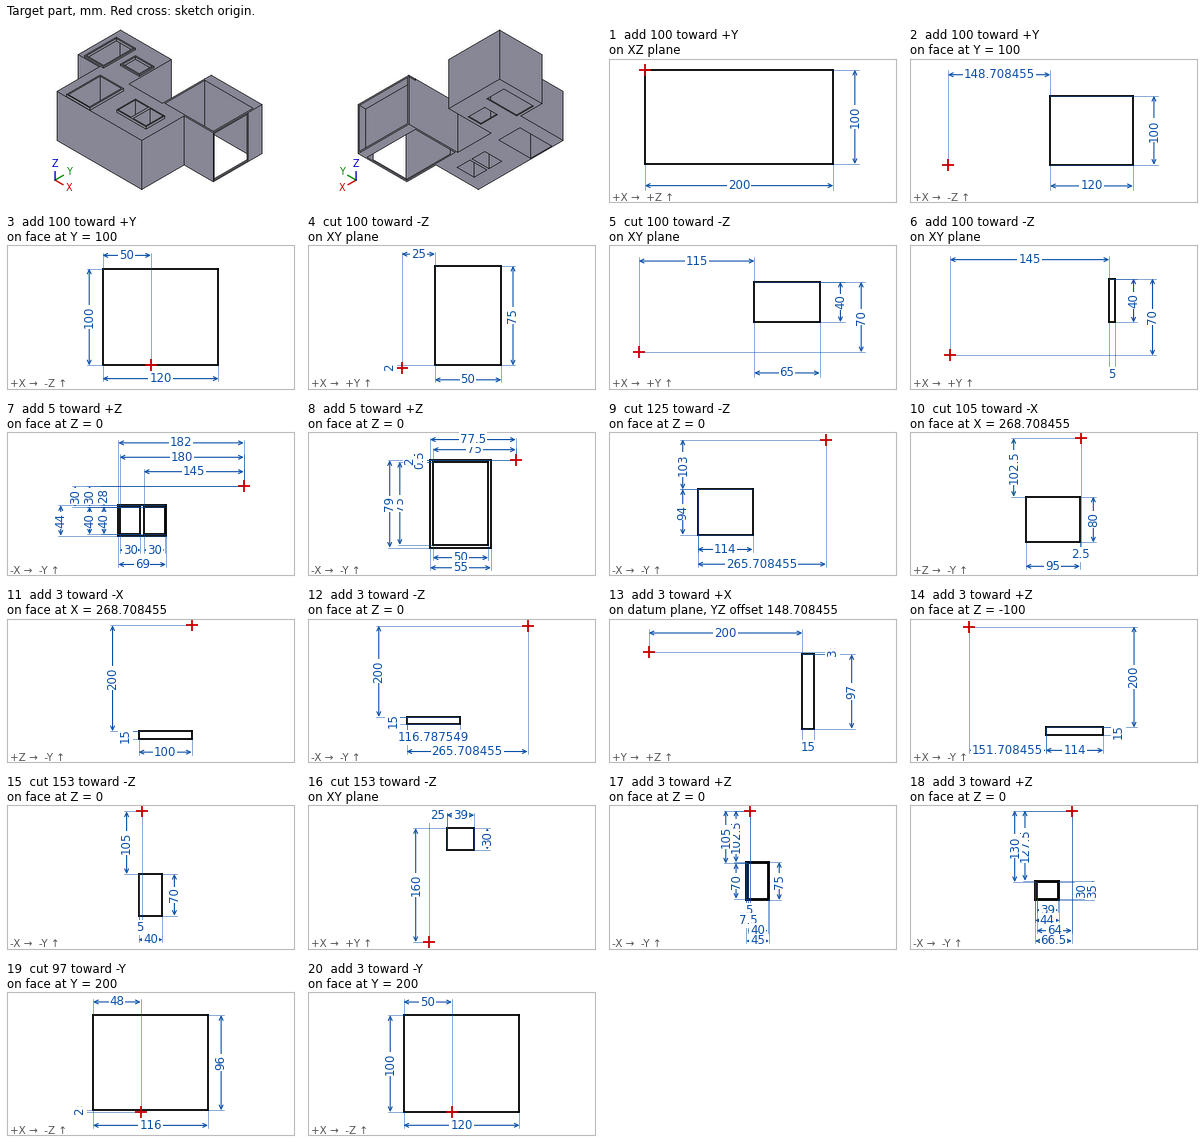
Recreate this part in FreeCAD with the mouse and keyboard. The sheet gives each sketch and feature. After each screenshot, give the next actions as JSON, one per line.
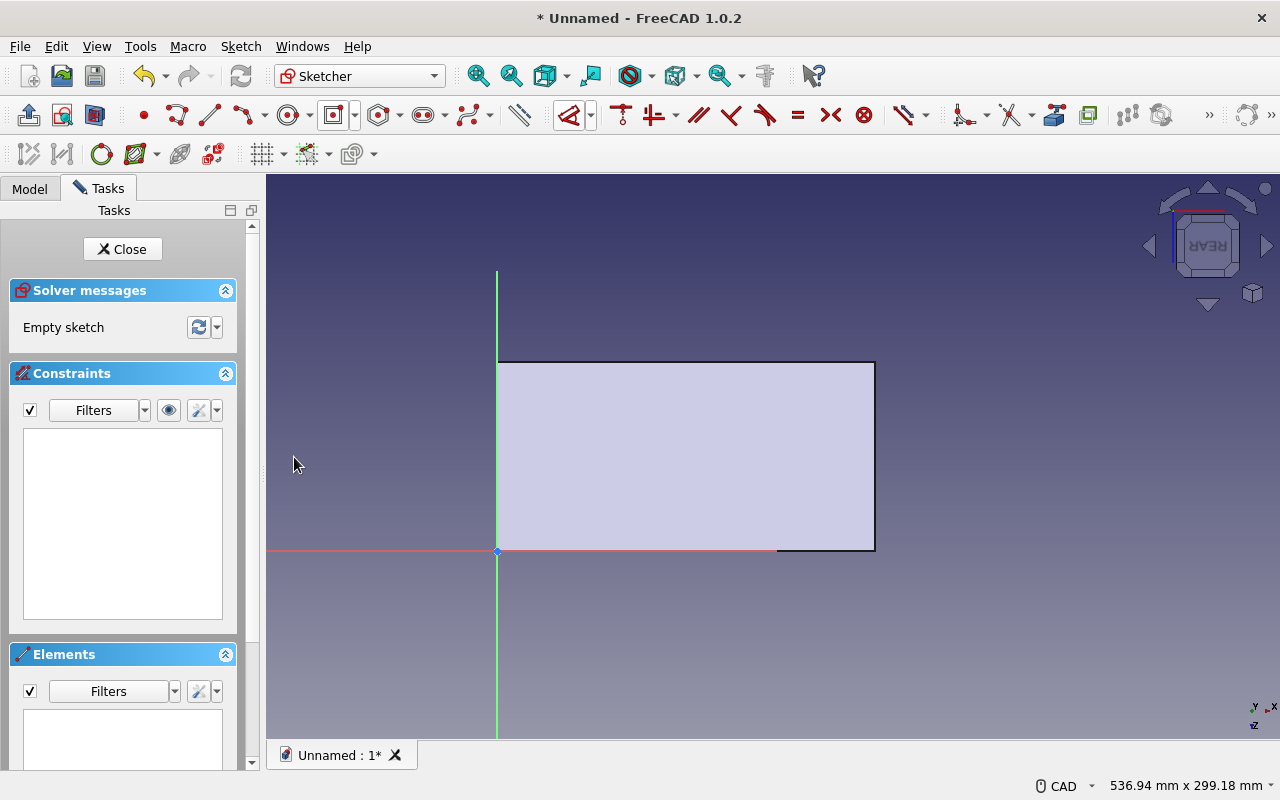
{"action": "key", "text": "g r"}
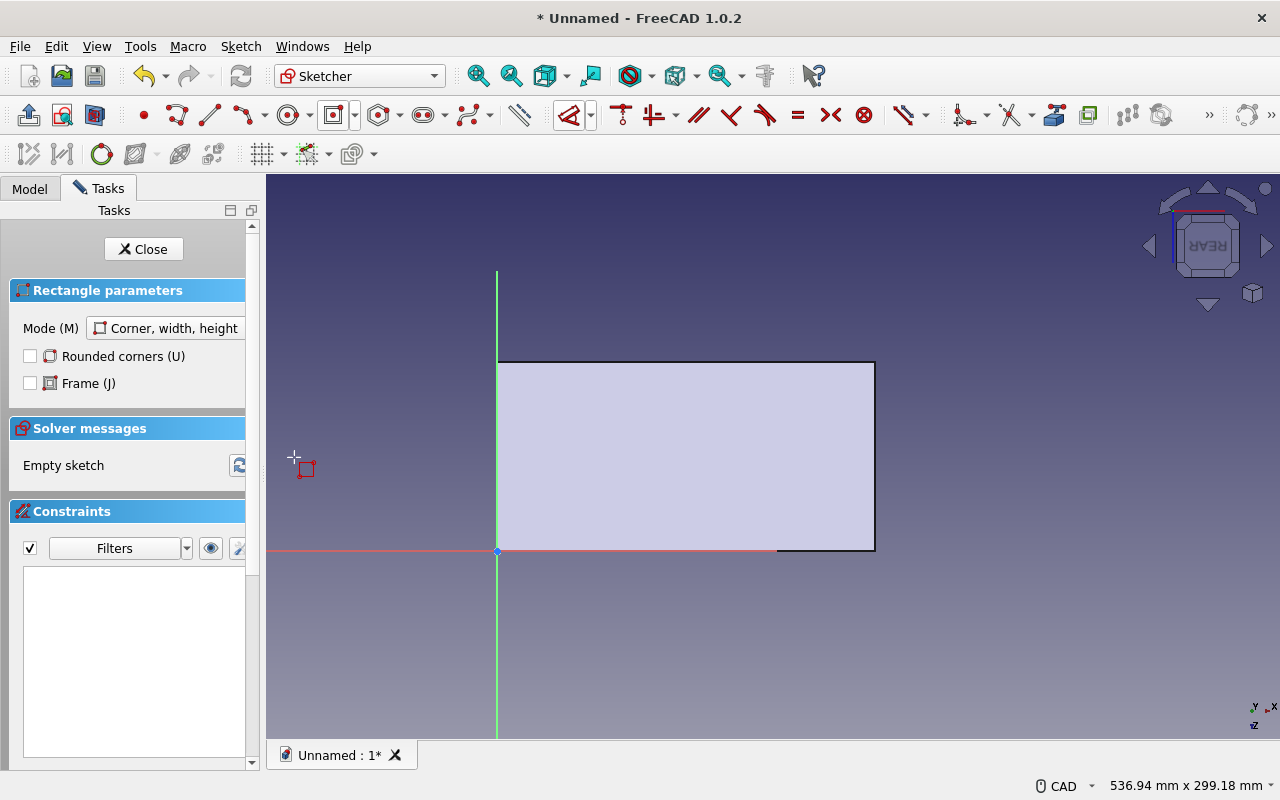
{"action": "left_click", "coordinate": [778, 362]}
{"action": "left_click", "coordinate": [1005, 551]}
{"action": "key", "text": "Escape"}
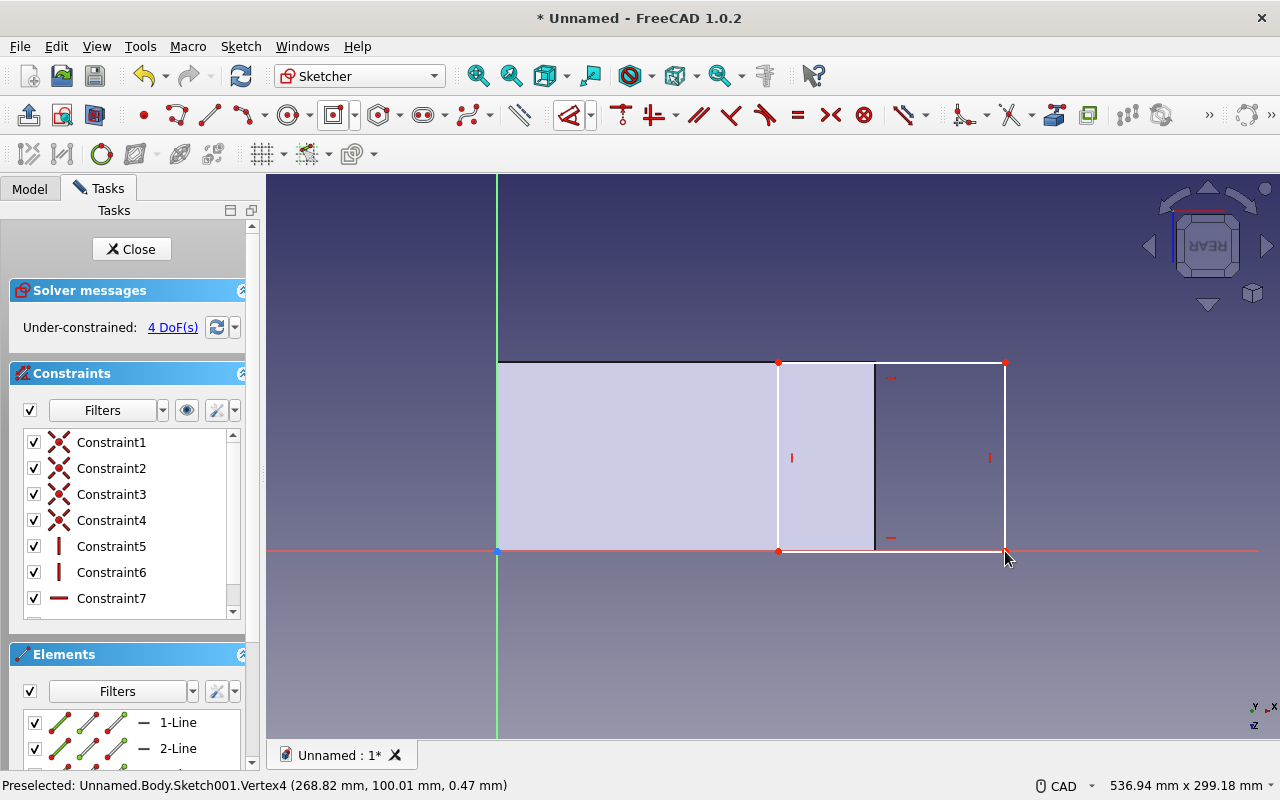
{"action": "left_click", "coordinate": [778, 552]}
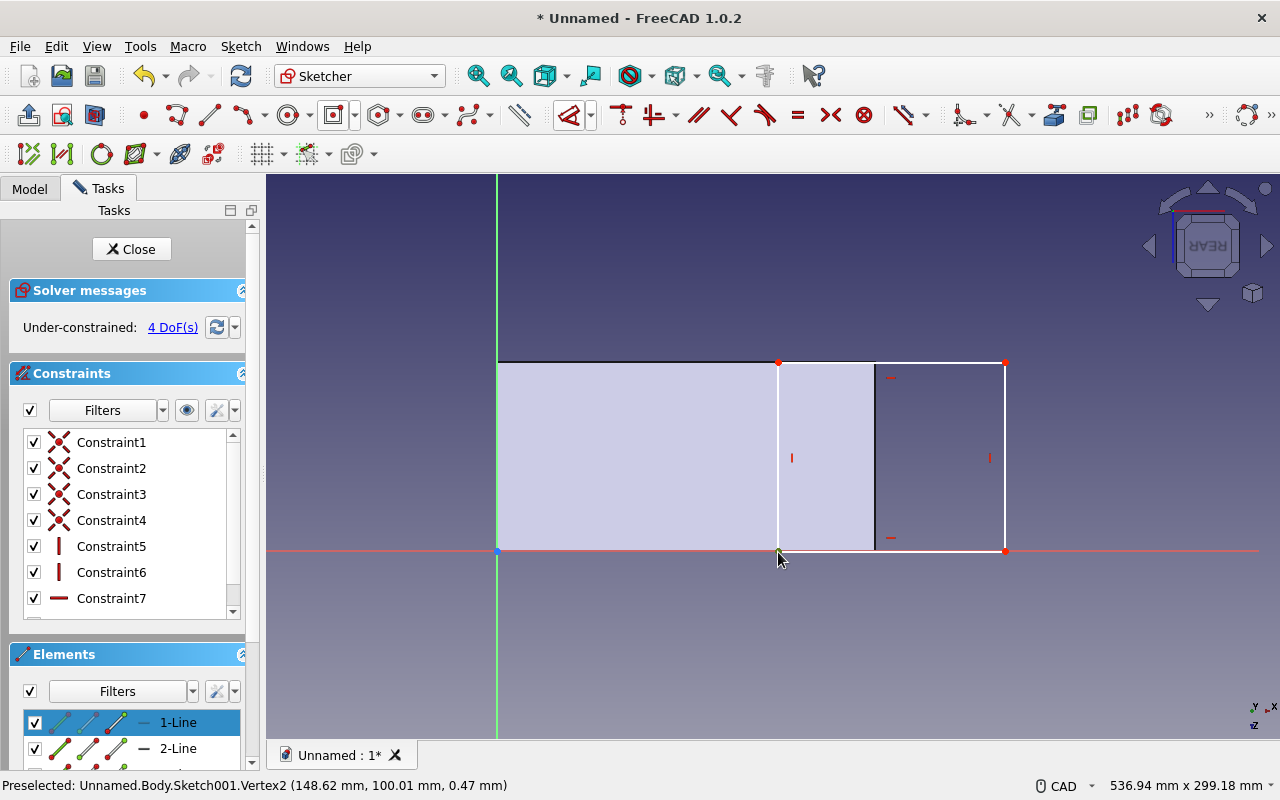
{"action": "left_click", "coordinate": [353, 551]}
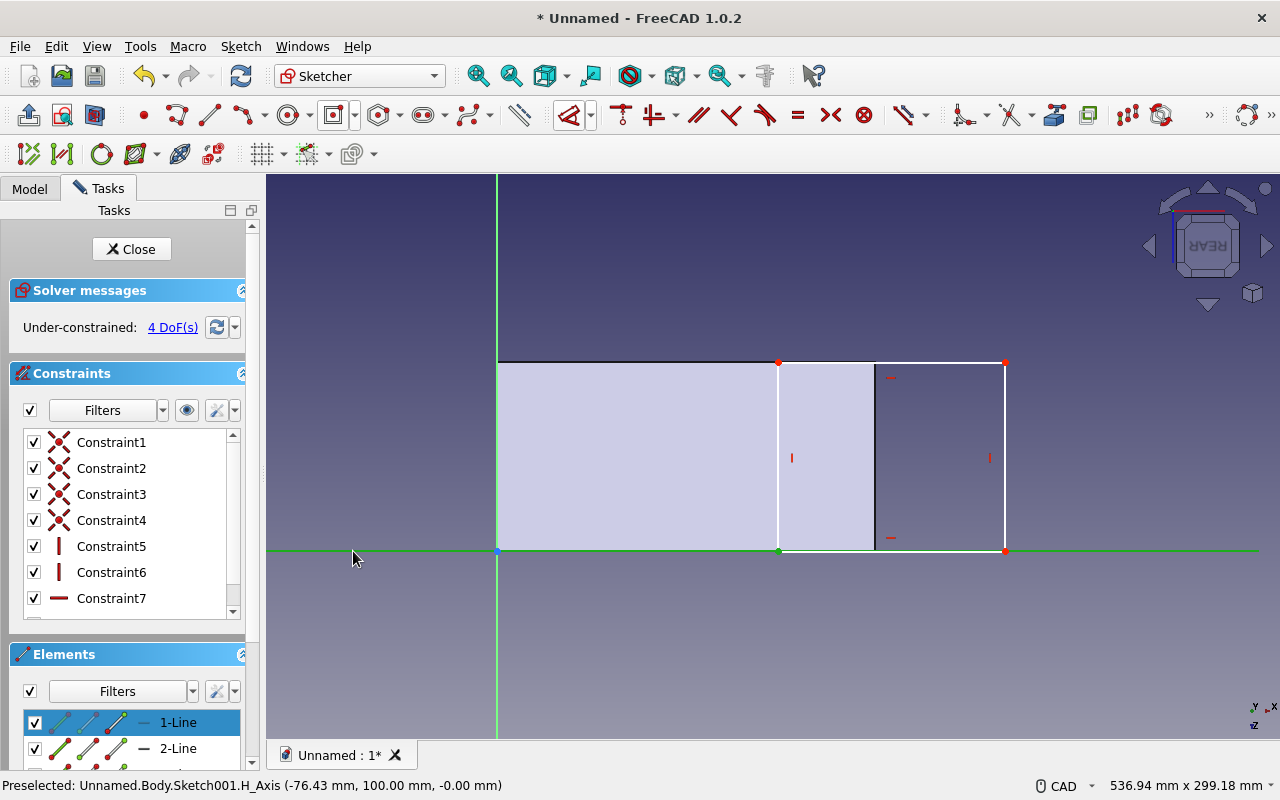
{"action": "left_click", "coordinate": [621, 116]}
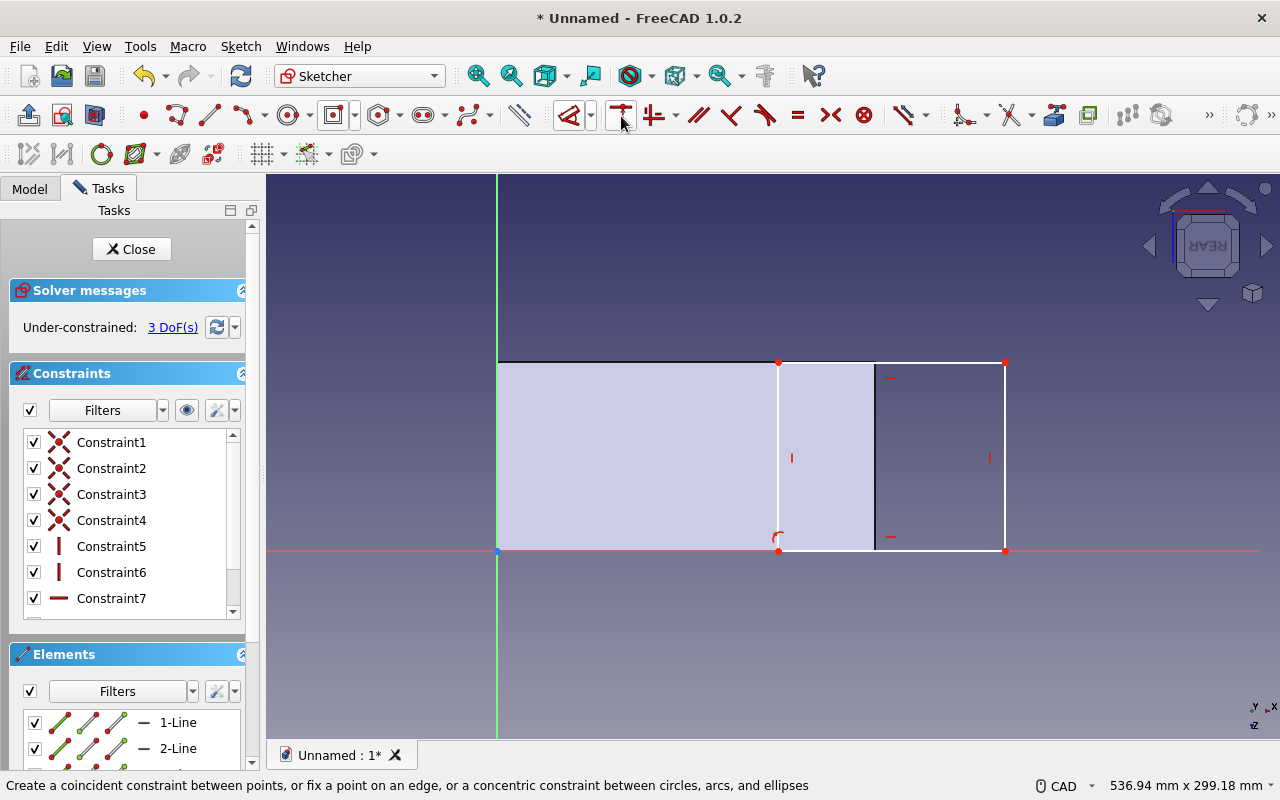
{"action": "left_click", "coordinate": [568, 116]}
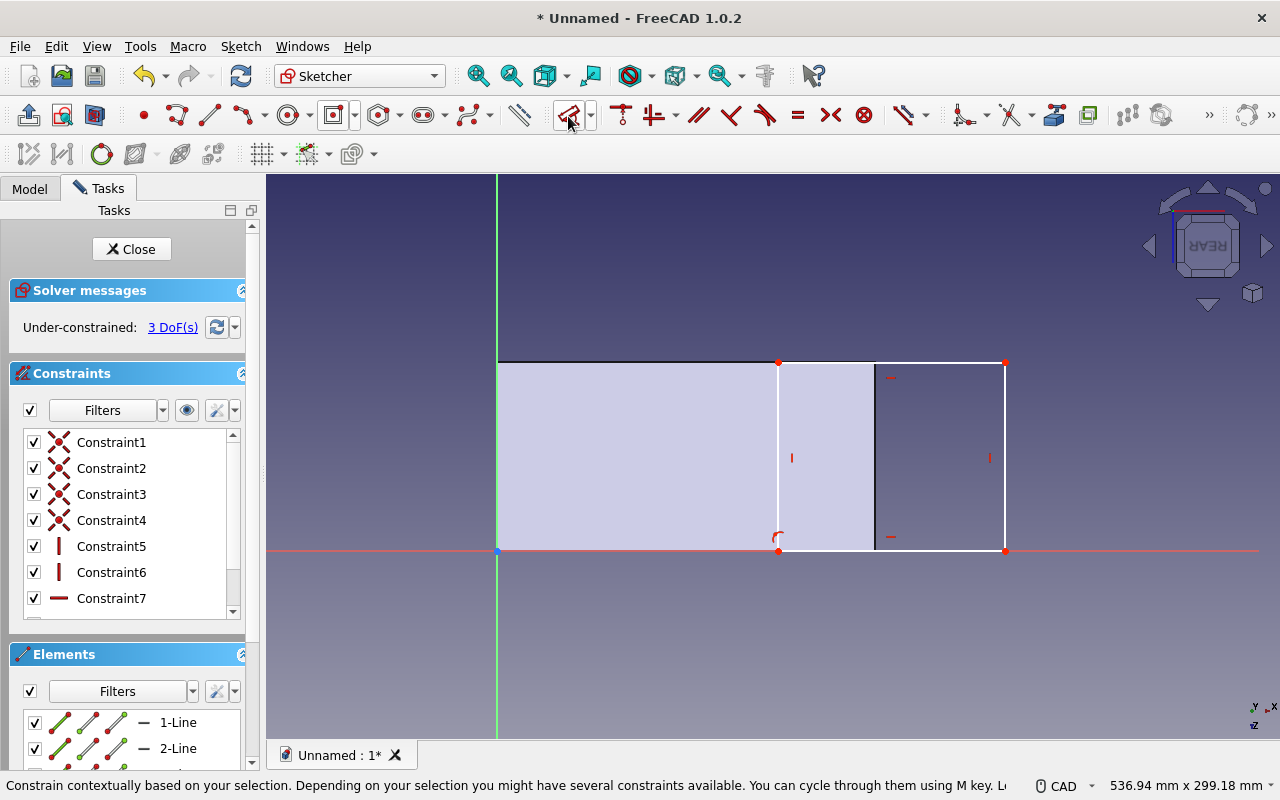
{"action": "left_click", "coordinate": [778, 419]}
{"action": "left_click", "coordinate": [812, 457]}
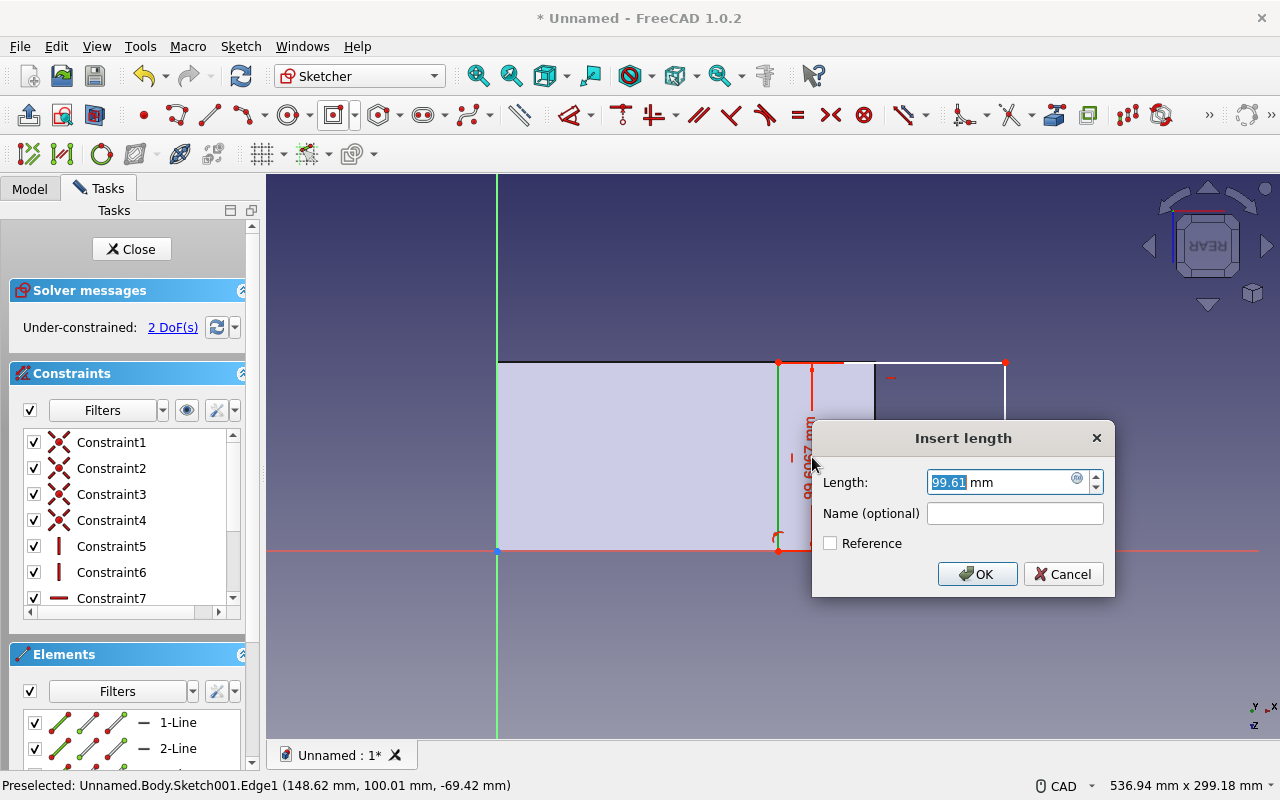
{"action": "type", "text": "100"}
{"action": "key", "text": "Return"}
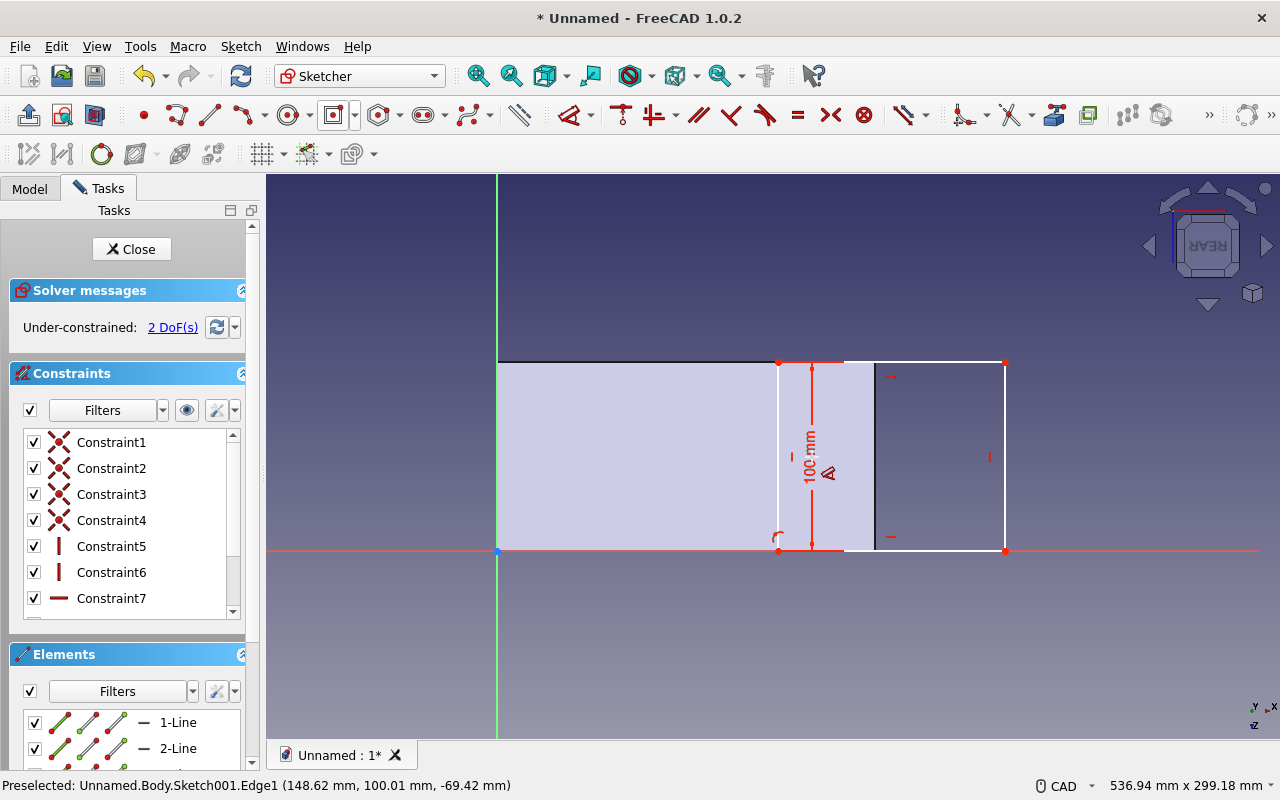
{"action": "left_click", "coordinate": [846, 551]}
{"action": "left_click", "coordinate": [892, 585]}